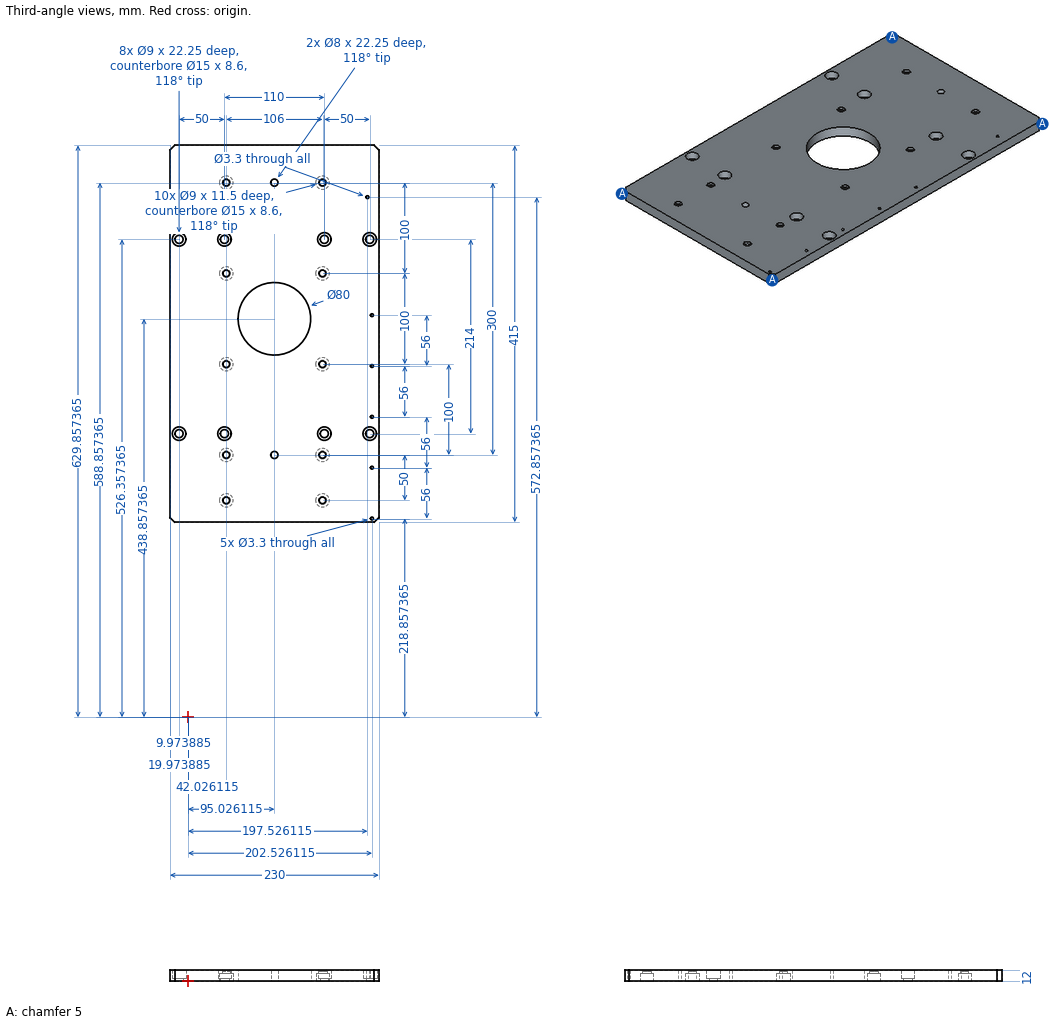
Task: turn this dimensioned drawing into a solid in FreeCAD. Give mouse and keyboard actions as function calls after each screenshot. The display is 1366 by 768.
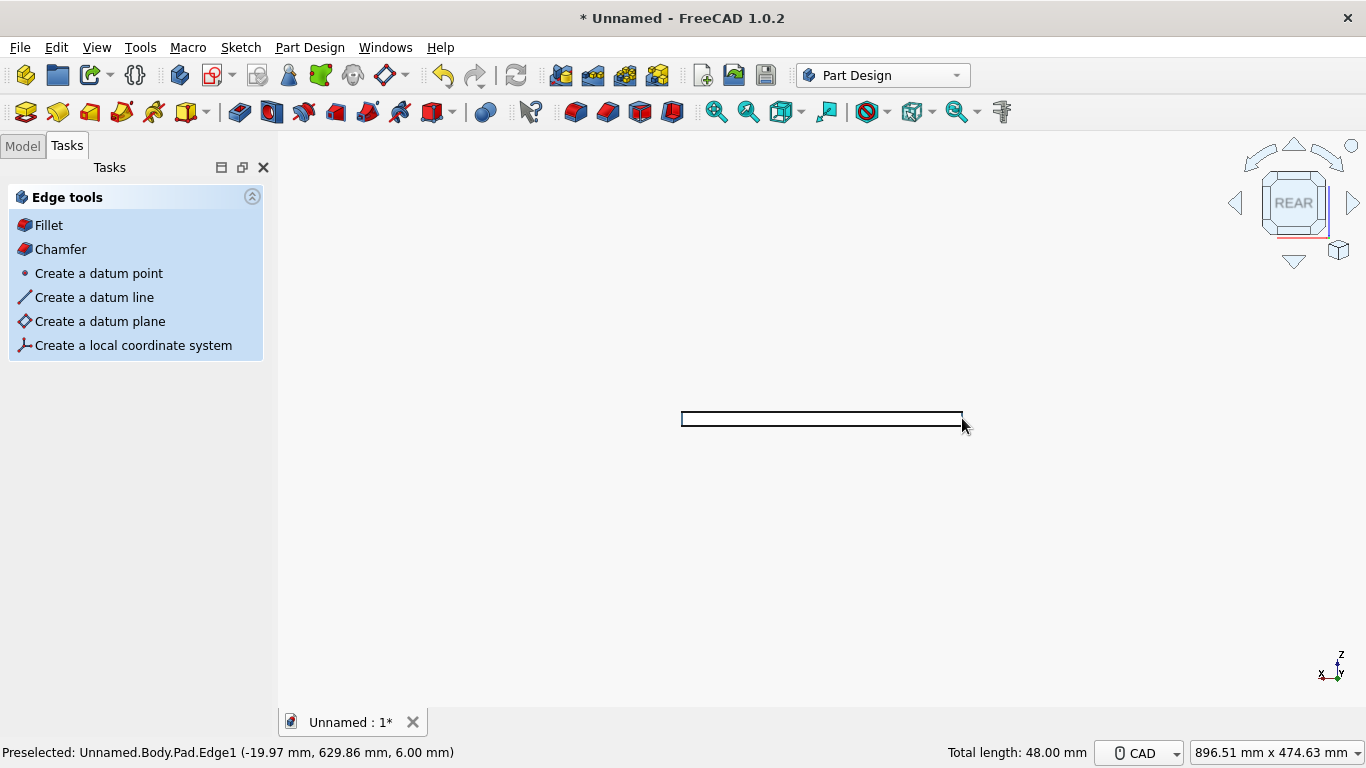
click(608, 112)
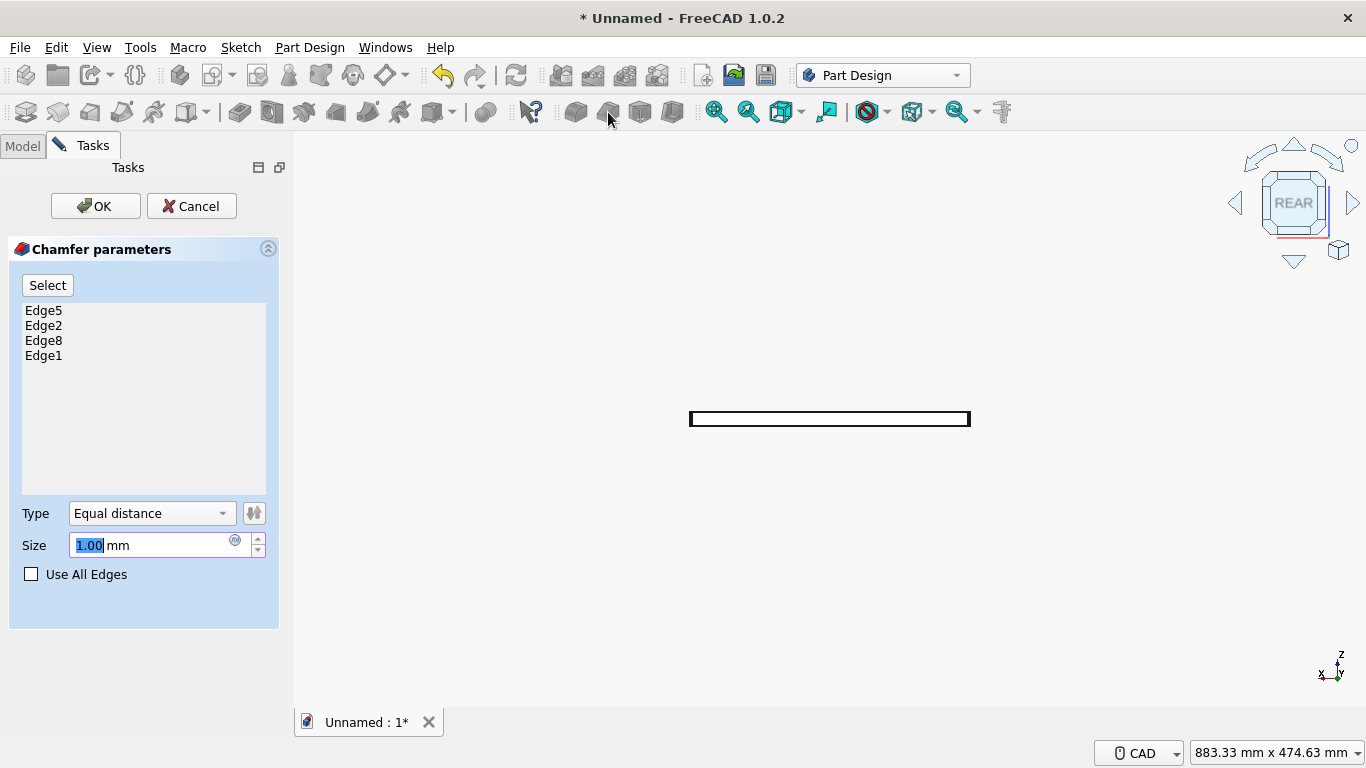
text(5)
key(Tab)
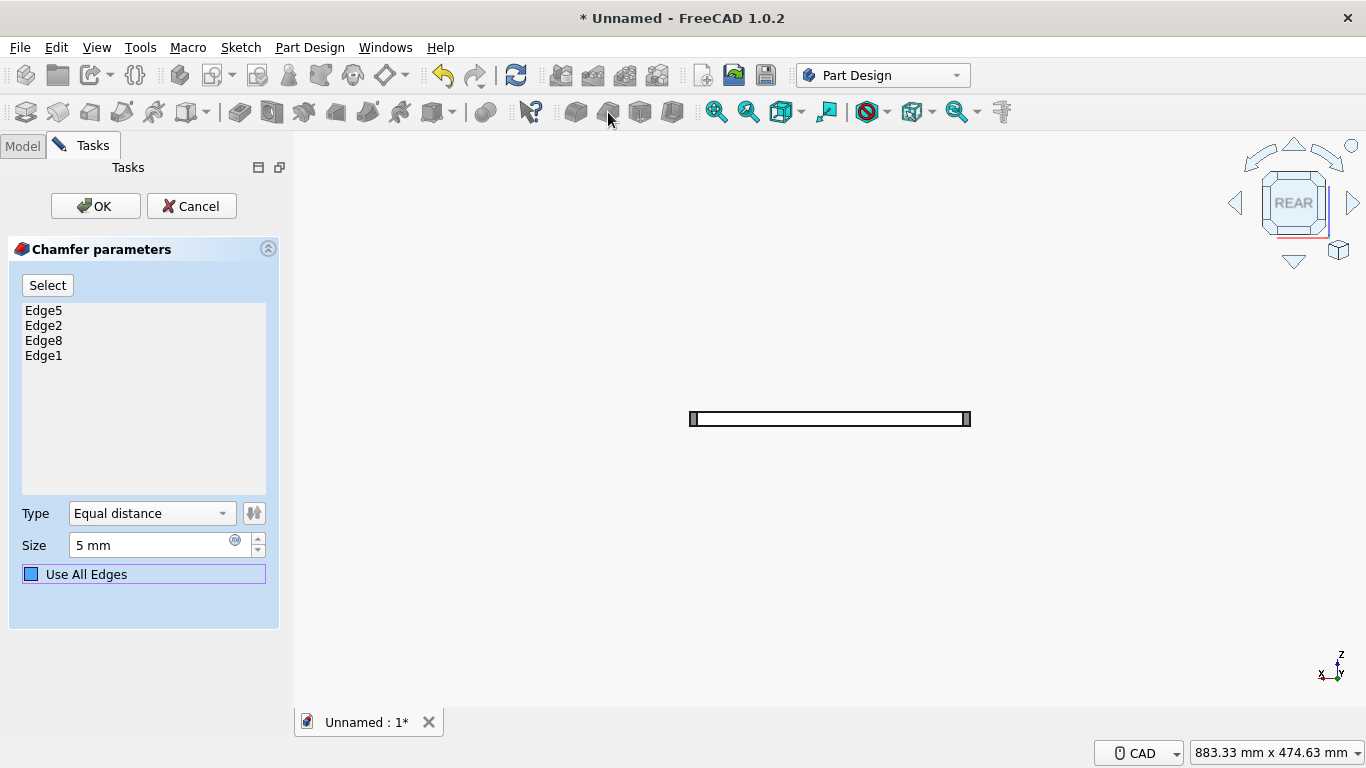
click(96, 206)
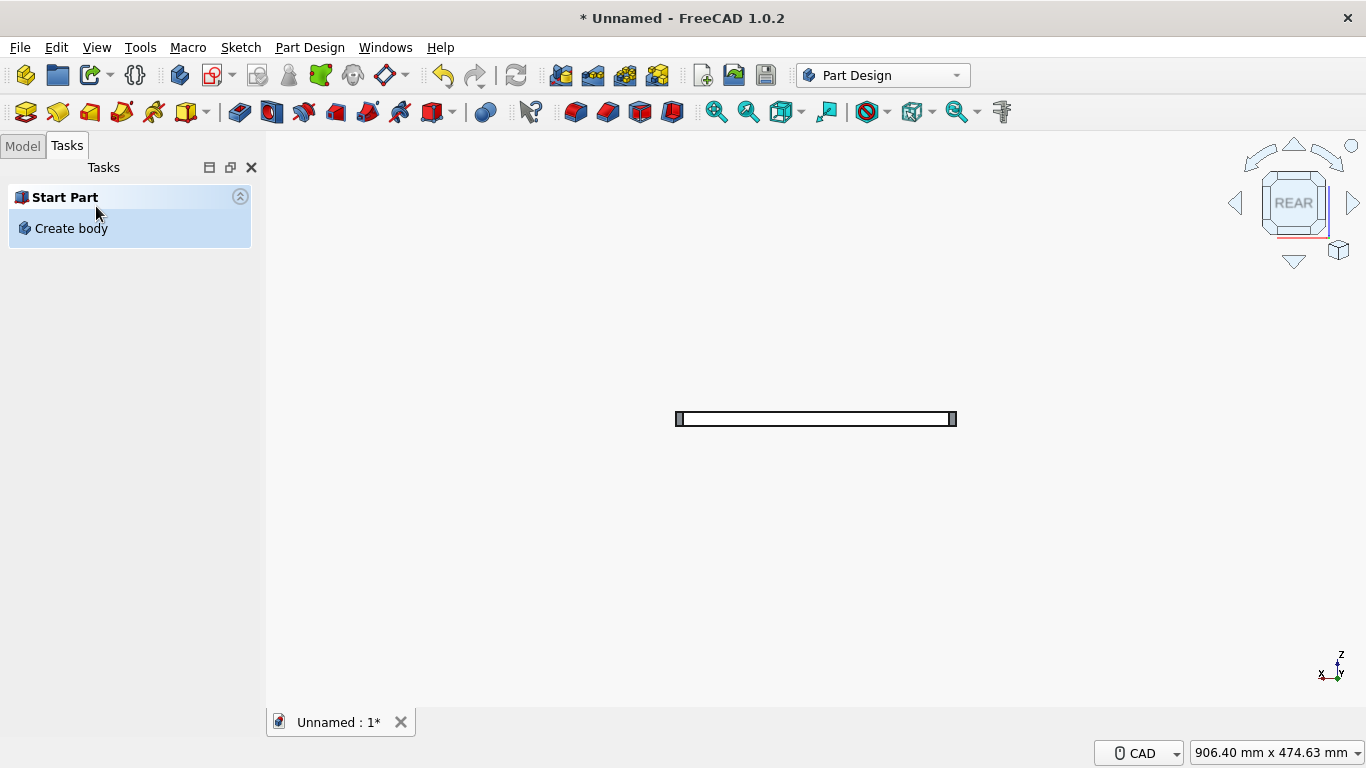
click(718, 112)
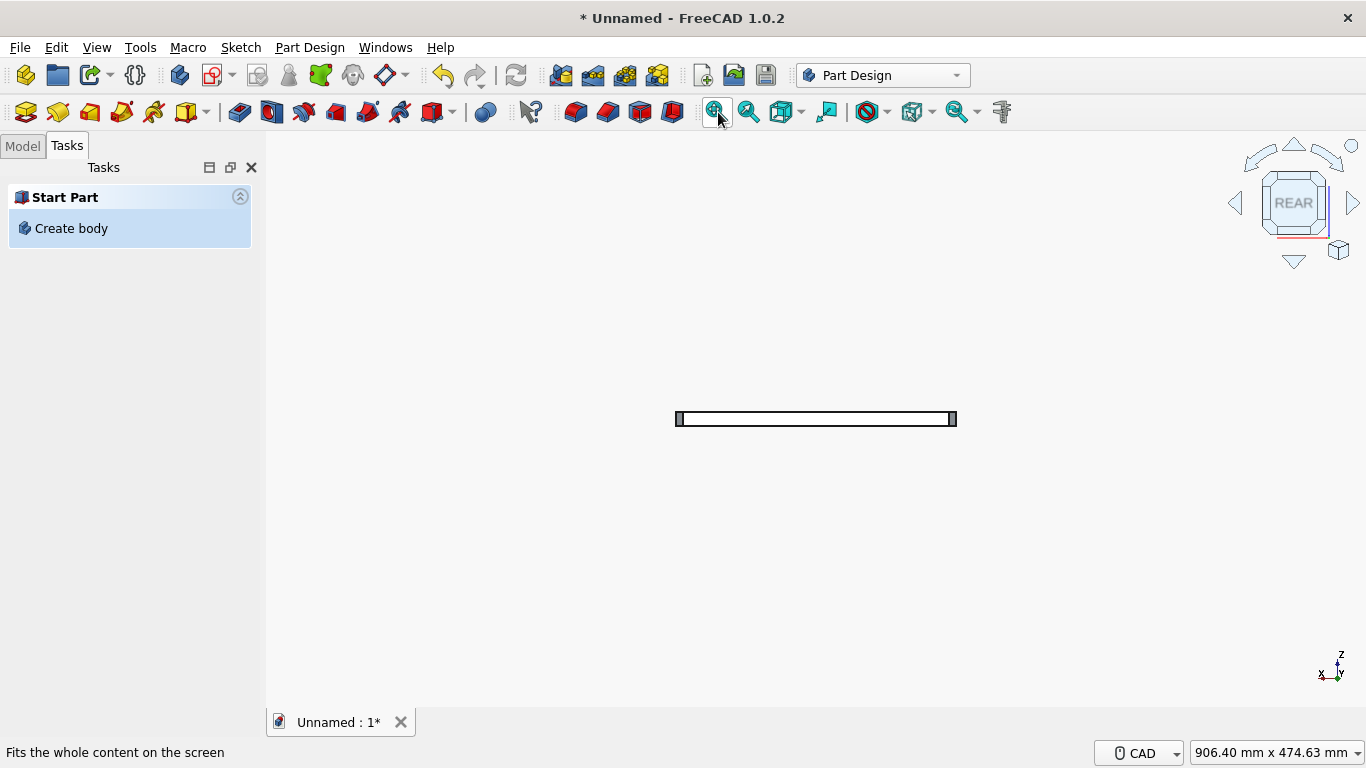
key(5)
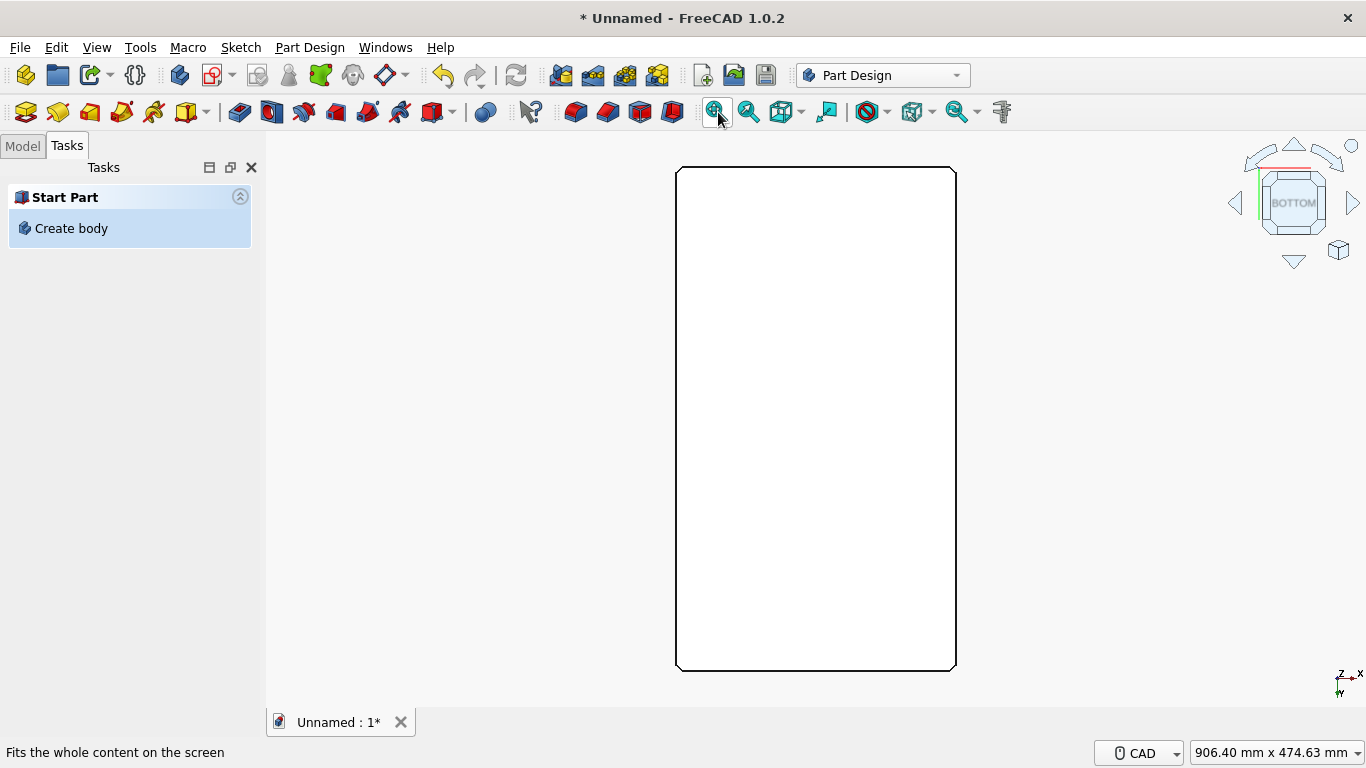
click(816, 490)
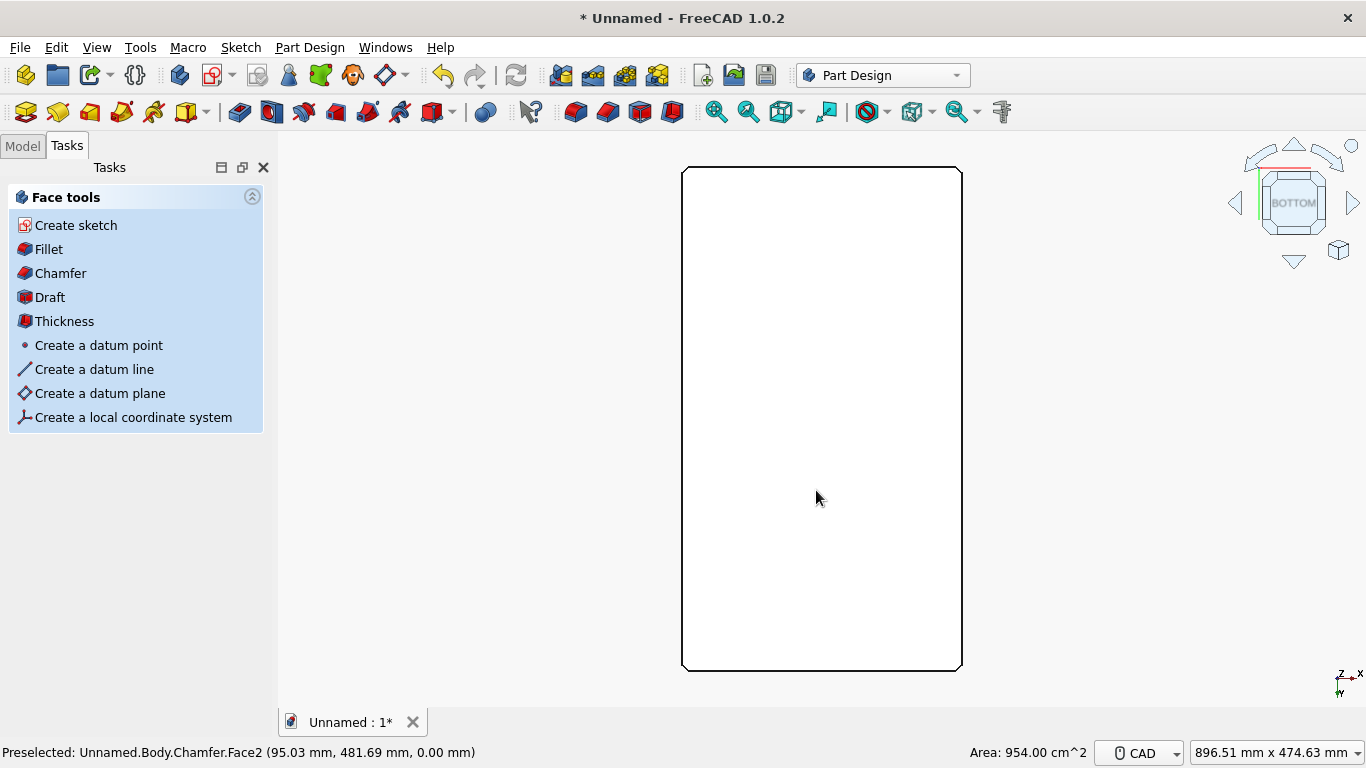
click(212, 76)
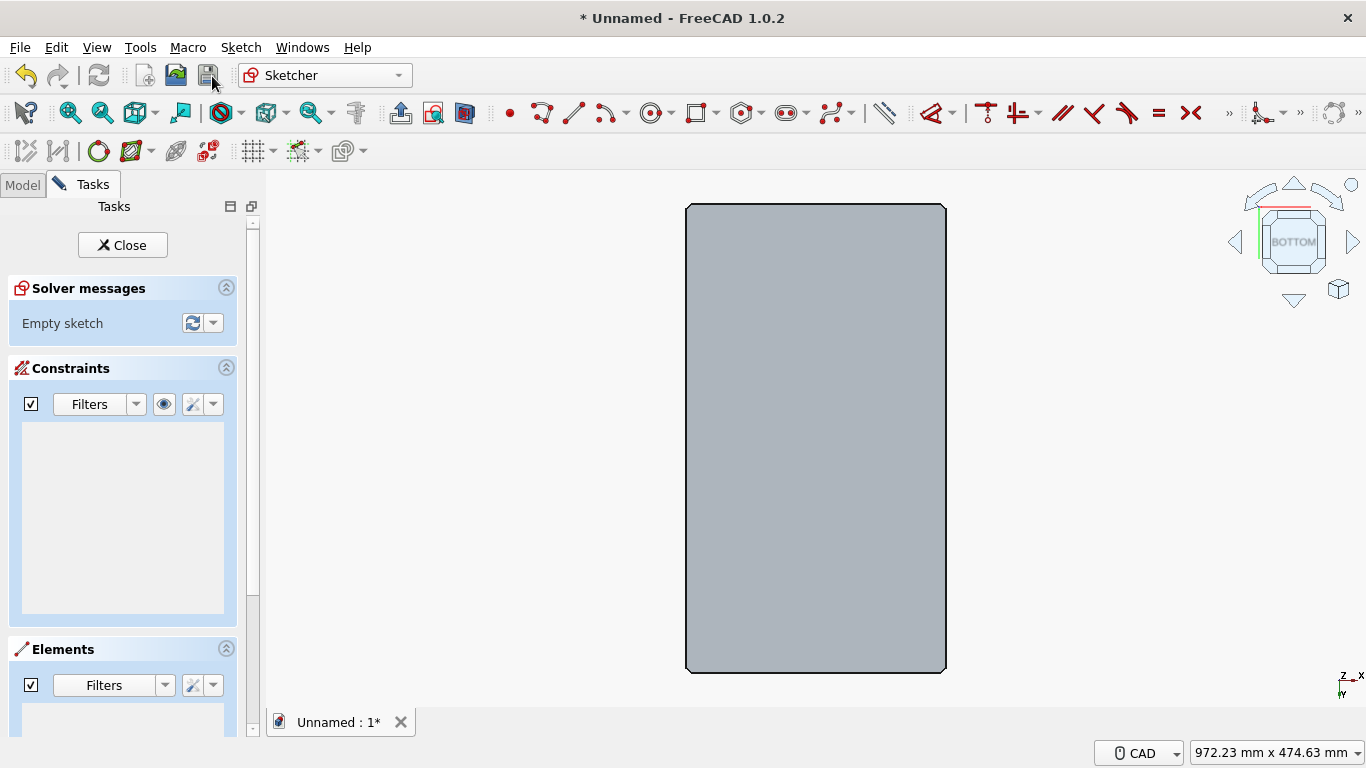
scroll(690, 611, down, 3)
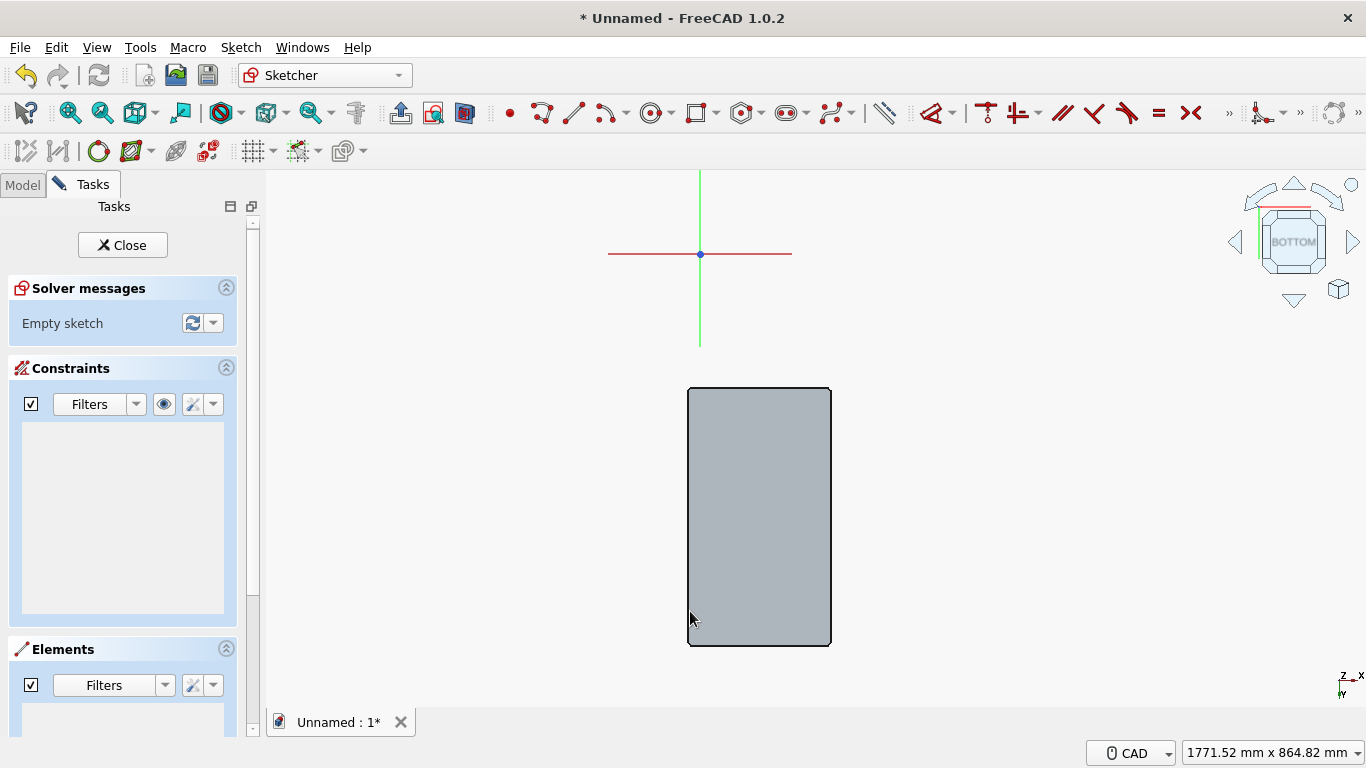
click(652, 114)